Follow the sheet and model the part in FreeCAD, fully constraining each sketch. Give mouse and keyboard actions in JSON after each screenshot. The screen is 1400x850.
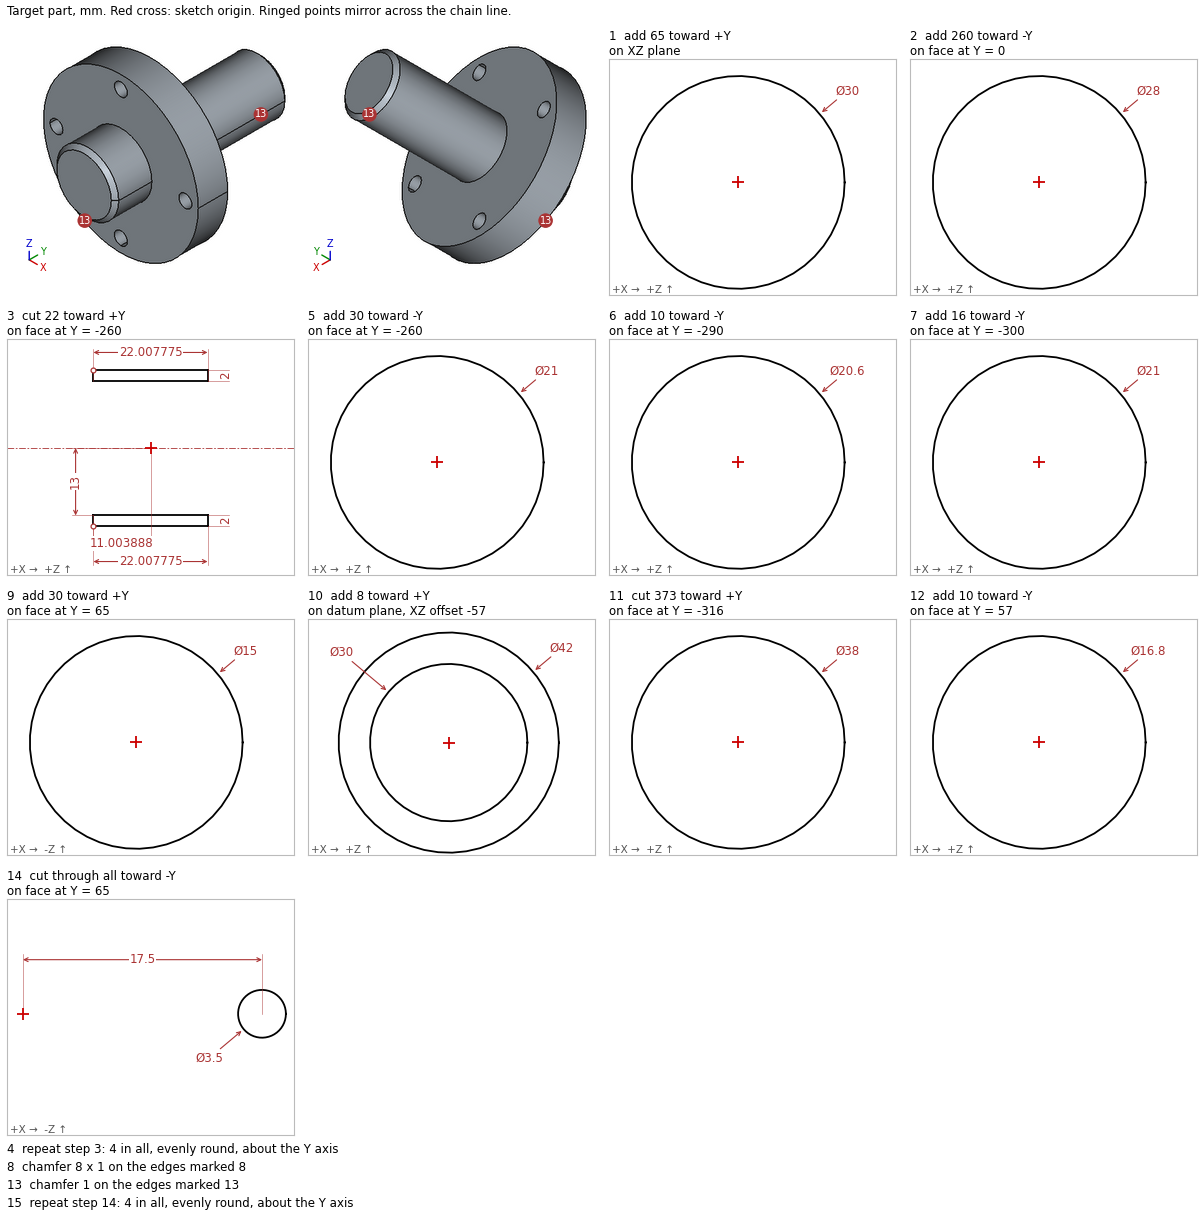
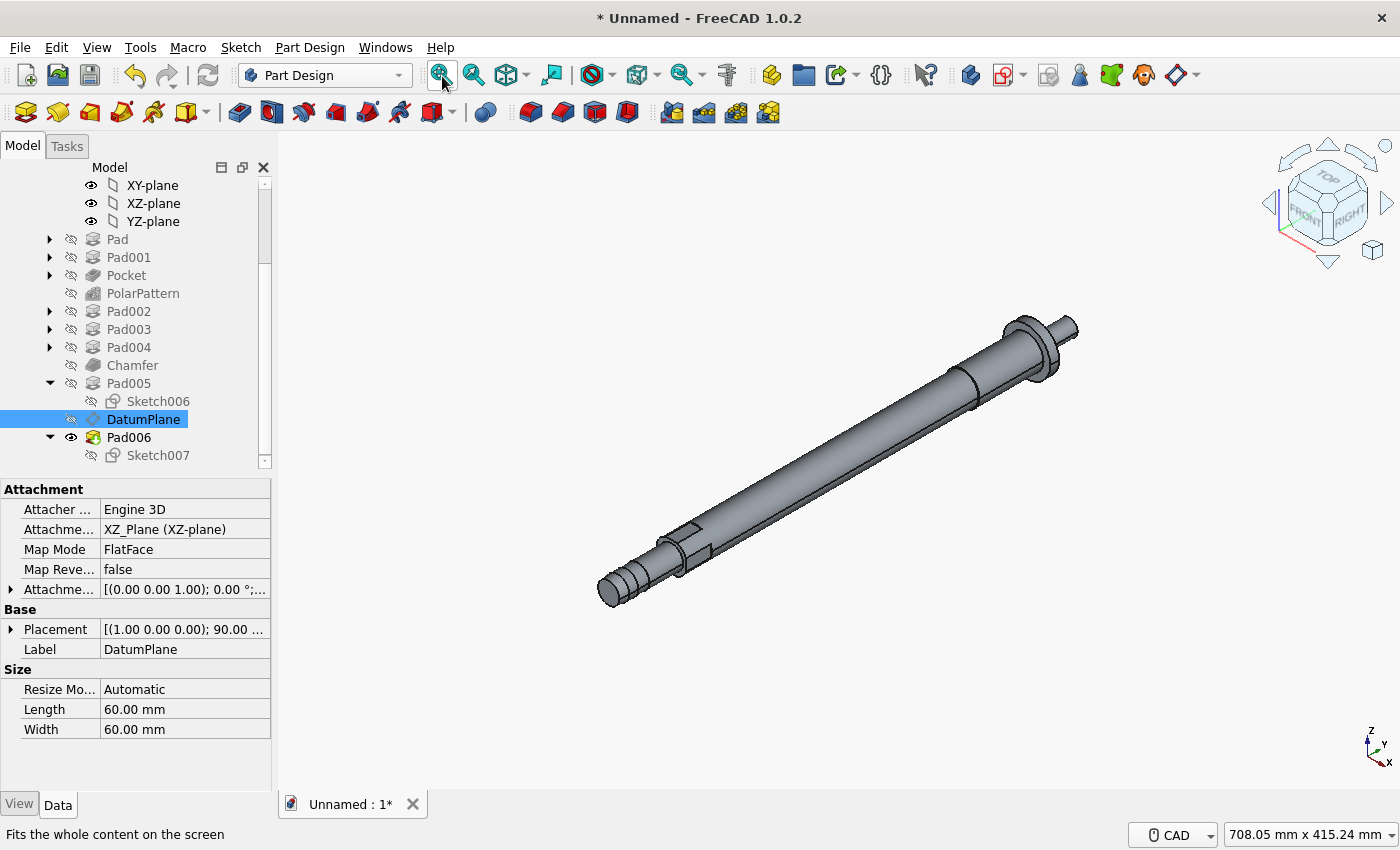
{"action": "left_click", "coordinate": [609, 595]}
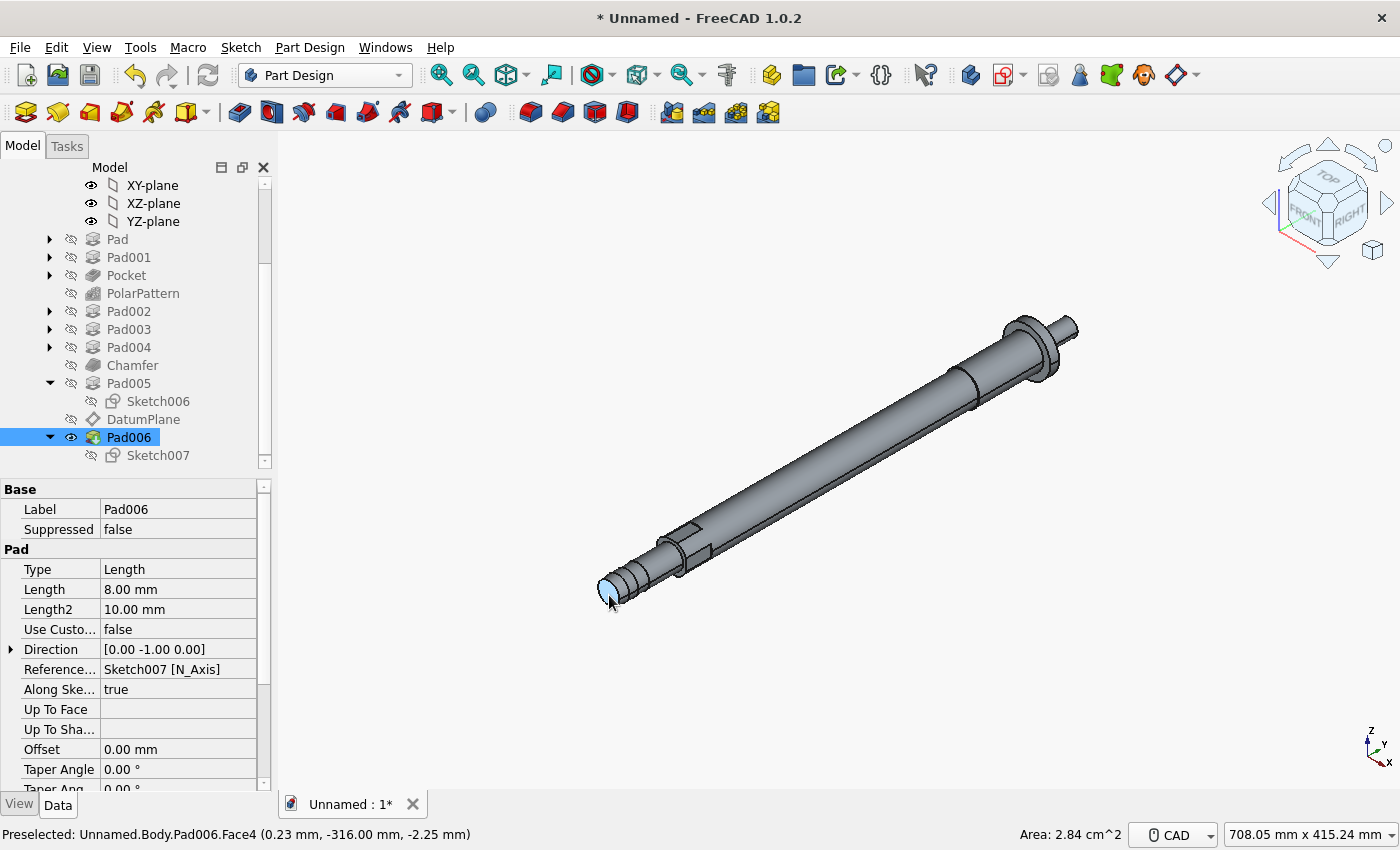
{"action": "left_click", "coordinate": [1004, 76]}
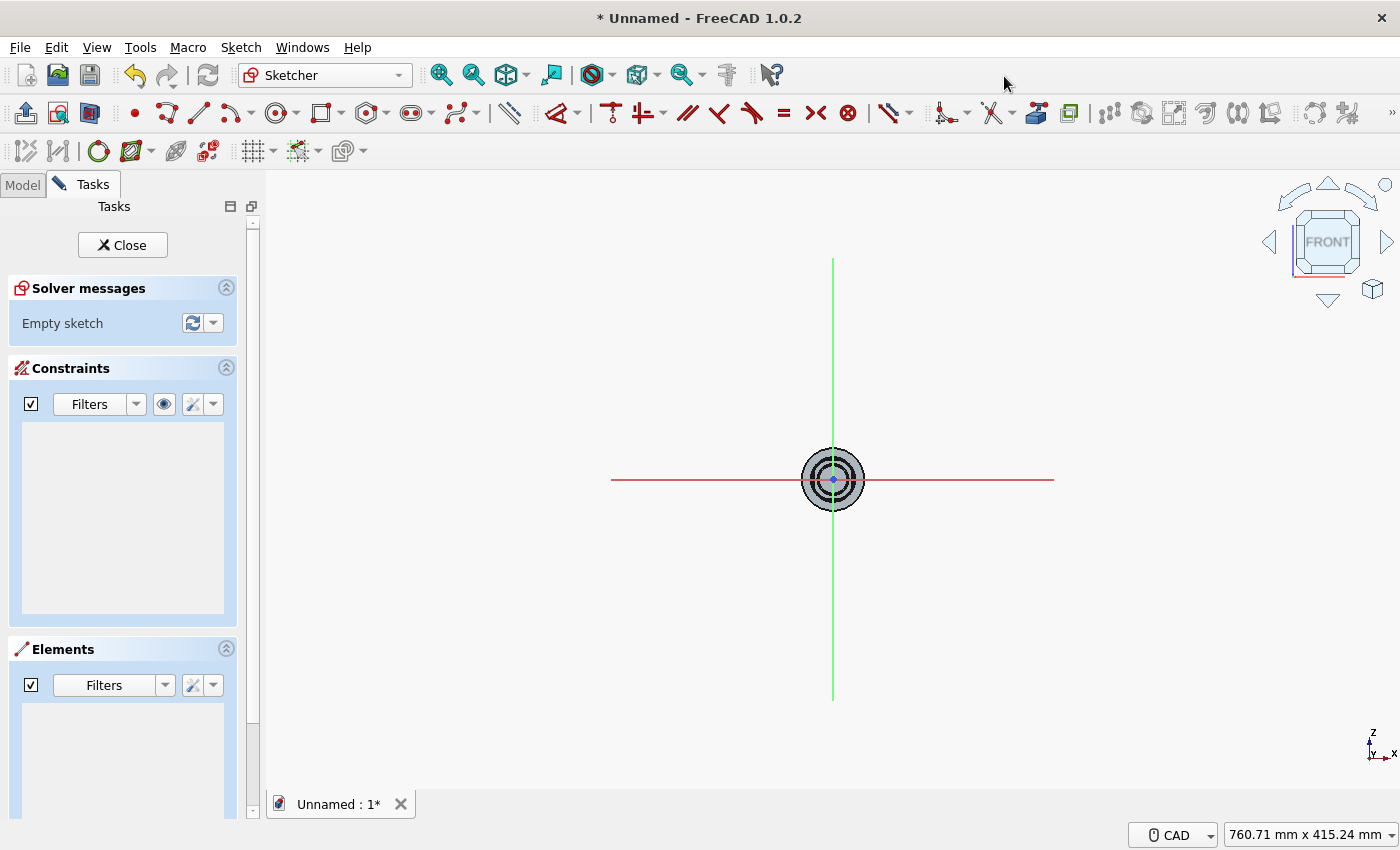
{"action": "scroll", "coordinate": [844, 480], "scroll_direction": "up", "scroll_amount": 10}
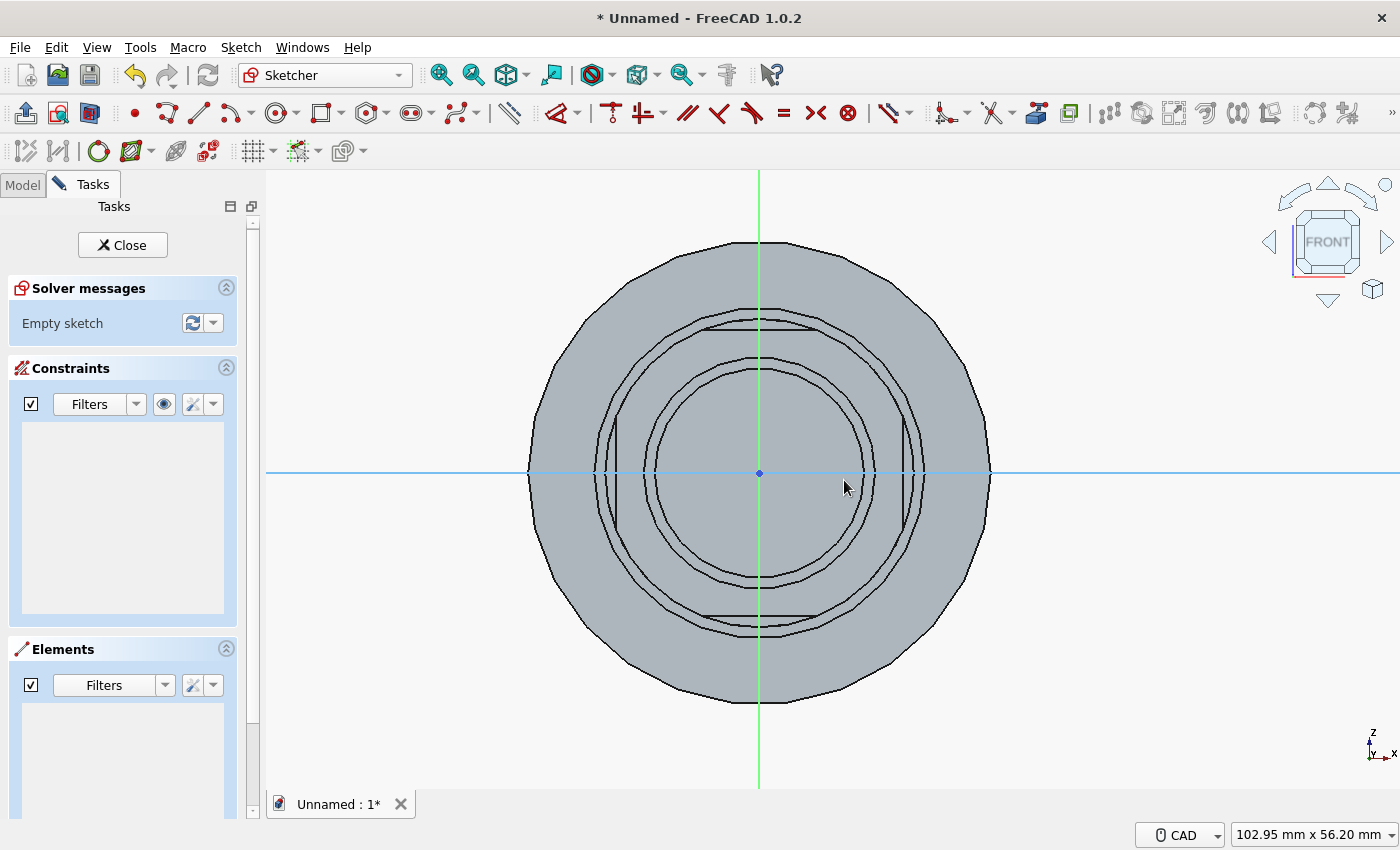
{"action": "left_click", "coordinate": [276, 114]}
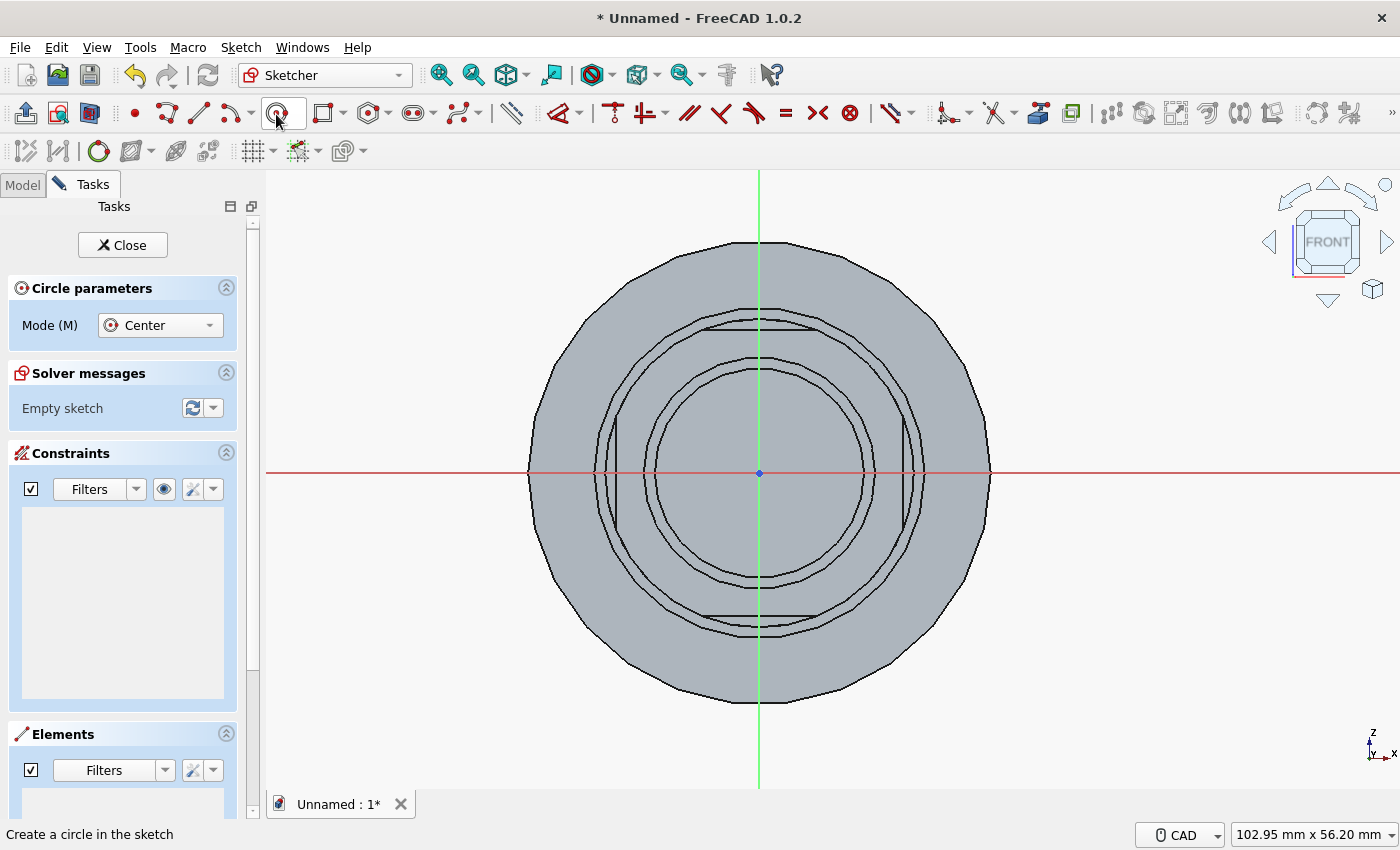
{"action": "left_click", "coordinate": [759, 473]}
{"action": "mouse_move", "coordinate": [907, 325]}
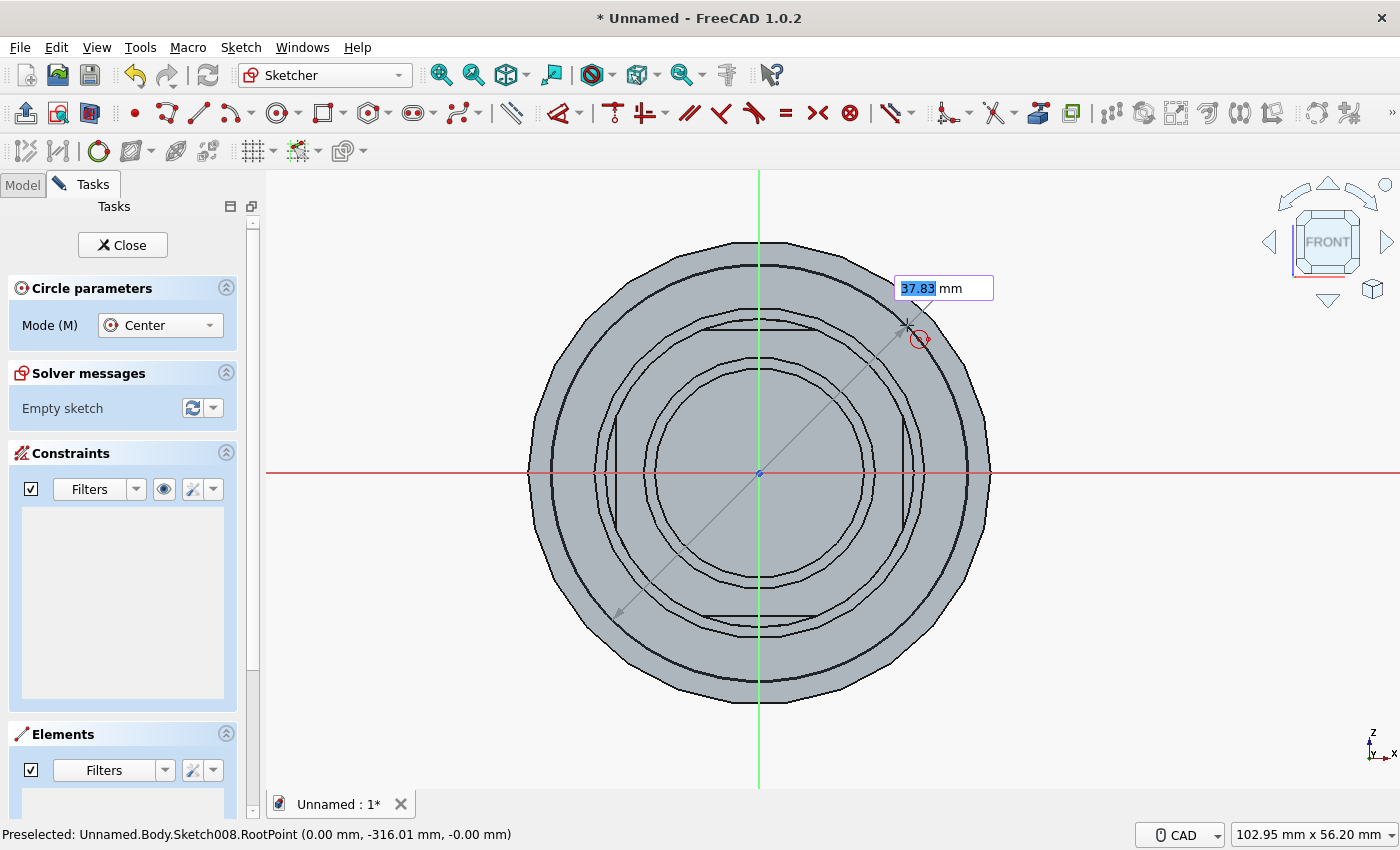
{"action": "type", "text": "38"}
{"action": "key", "text": "Return"}
{"action": "key", "text": "Escape"}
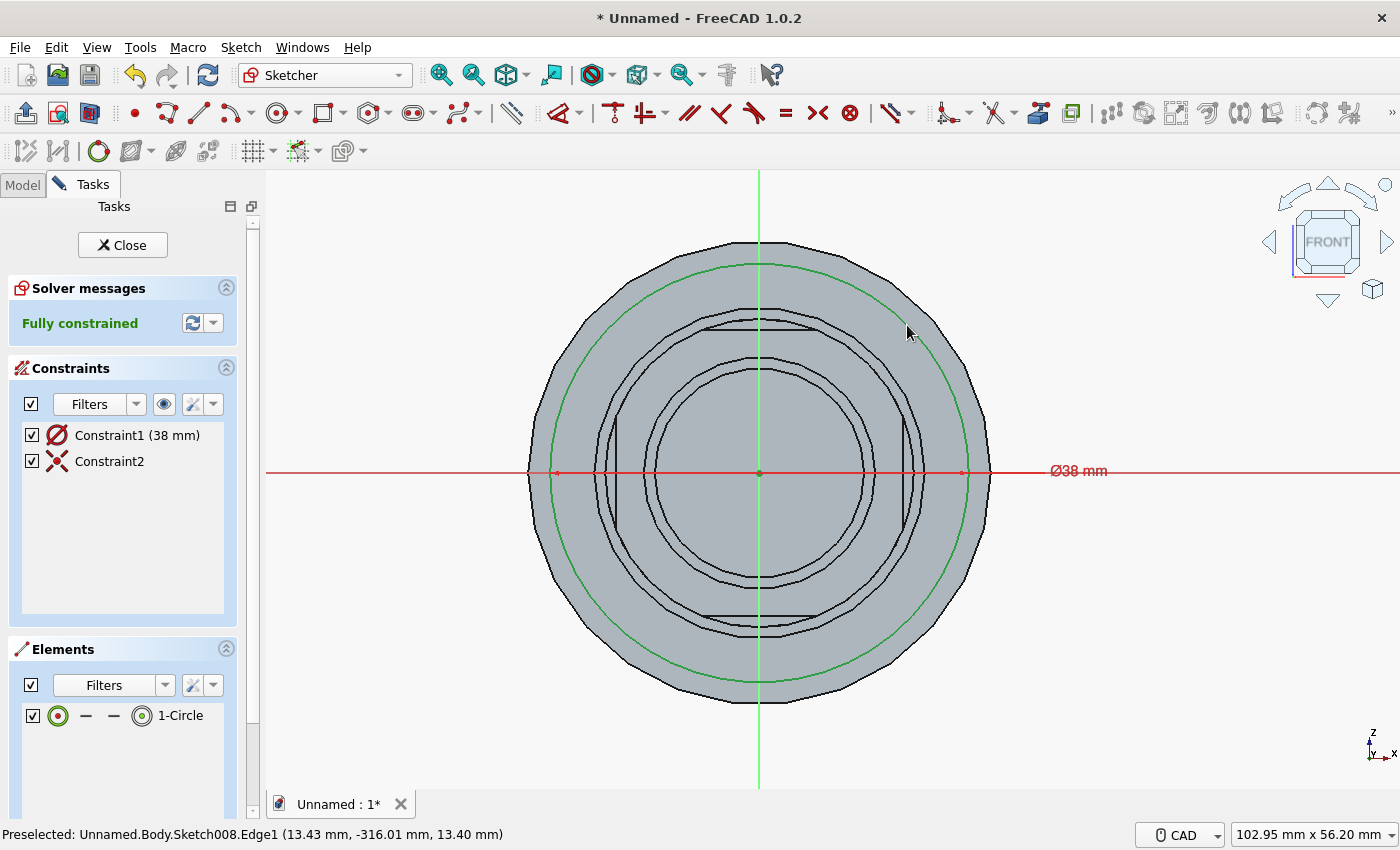
{"action": "left_click", "coordinate": [123, 245]}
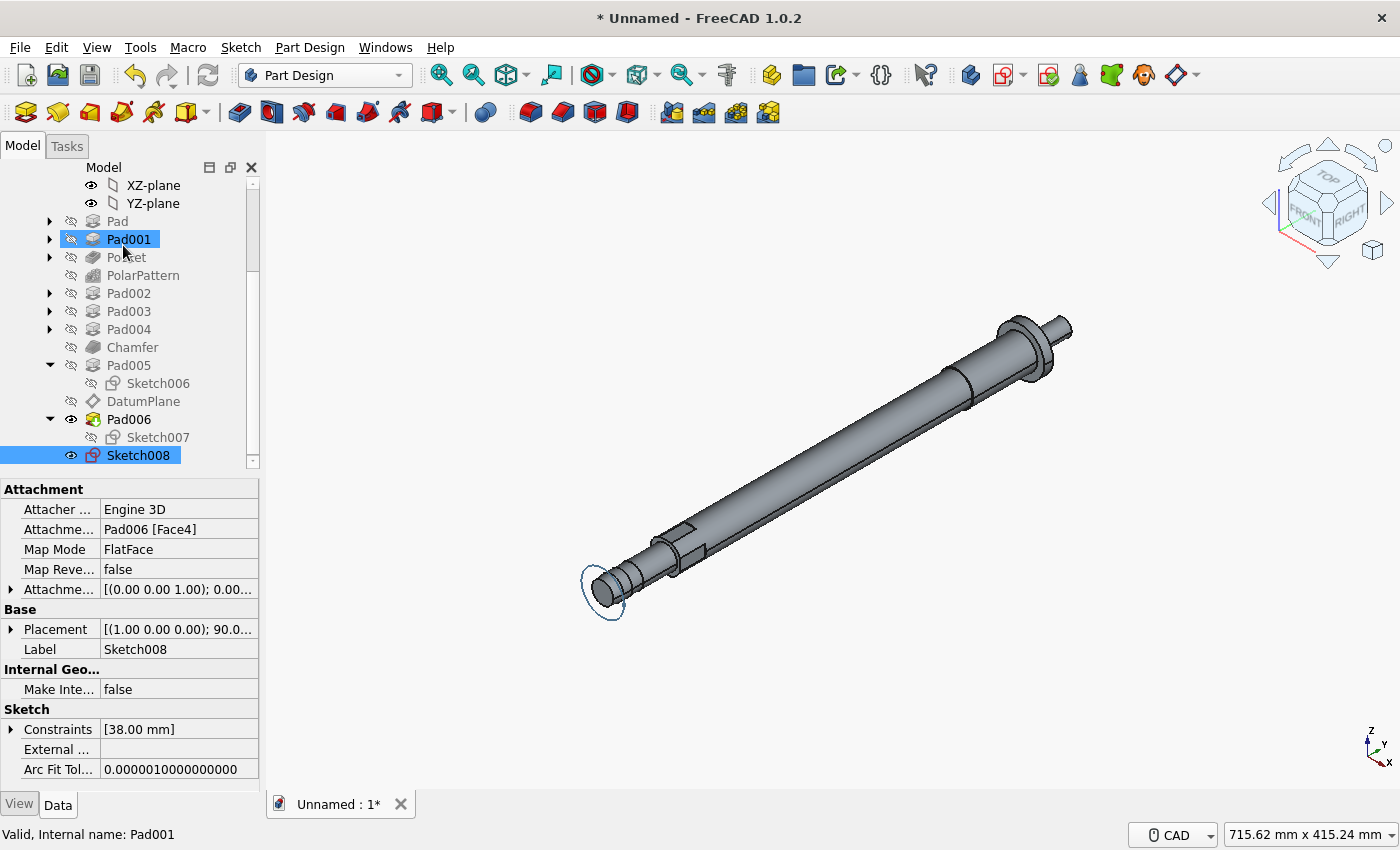
{"action": "left_click", "coordinate": [240, 112]}